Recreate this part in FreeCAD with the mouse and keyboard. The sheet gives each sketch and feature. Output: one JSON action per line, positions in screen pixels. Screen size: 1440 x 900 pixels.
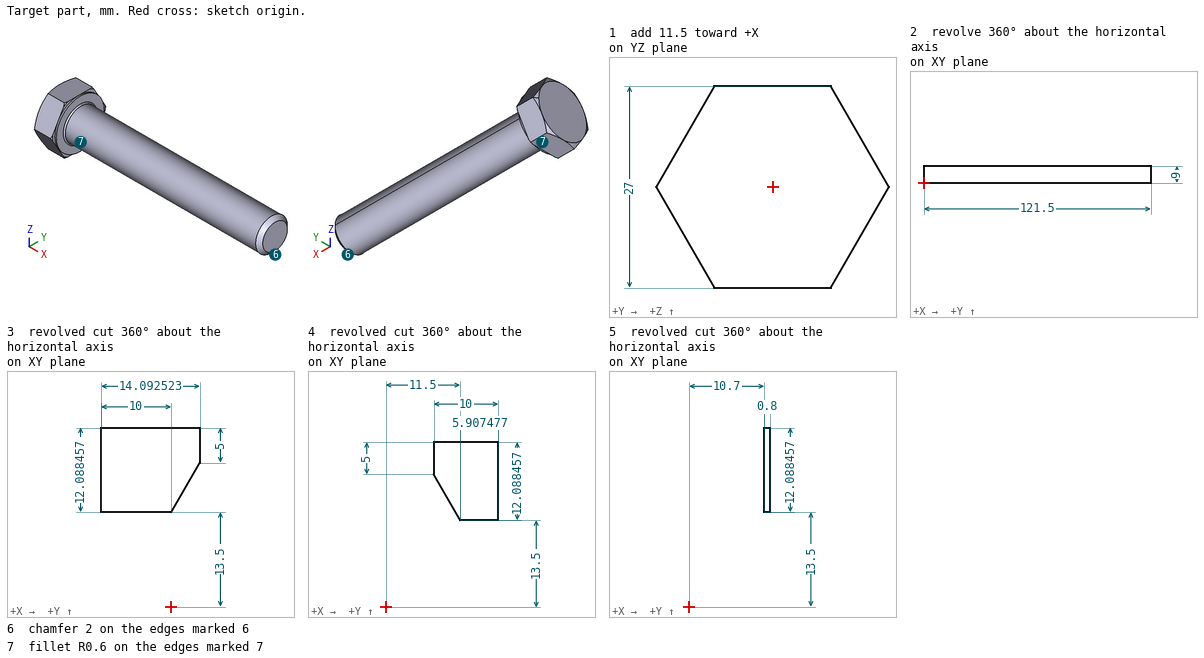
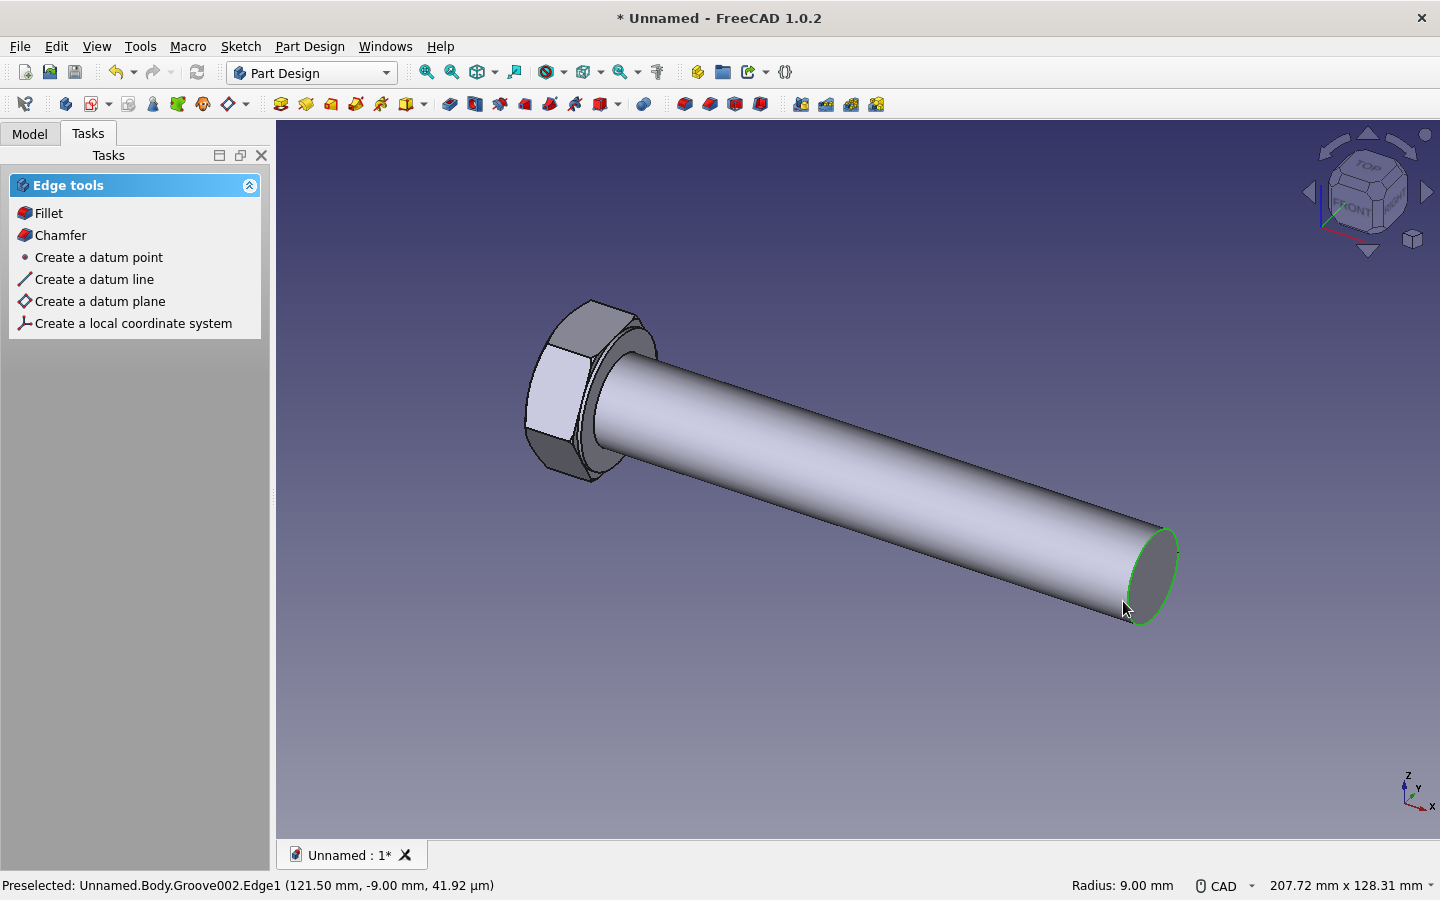
{"action": "left_click", "coordinate": [710, 104]}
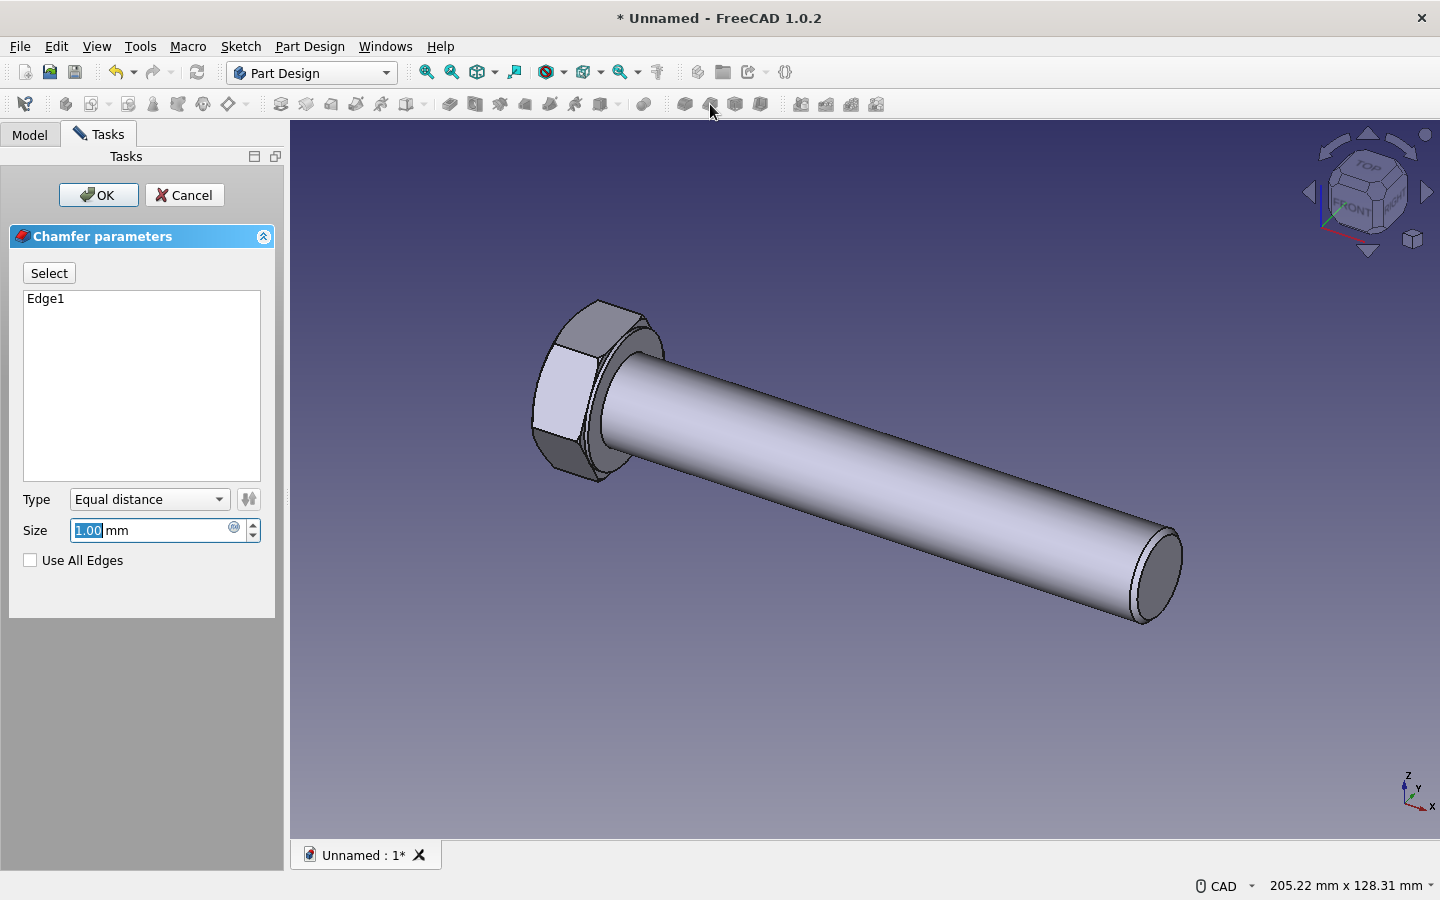
{"action": "type", "text": "2"}
{"action": "key", "text": "Tab"}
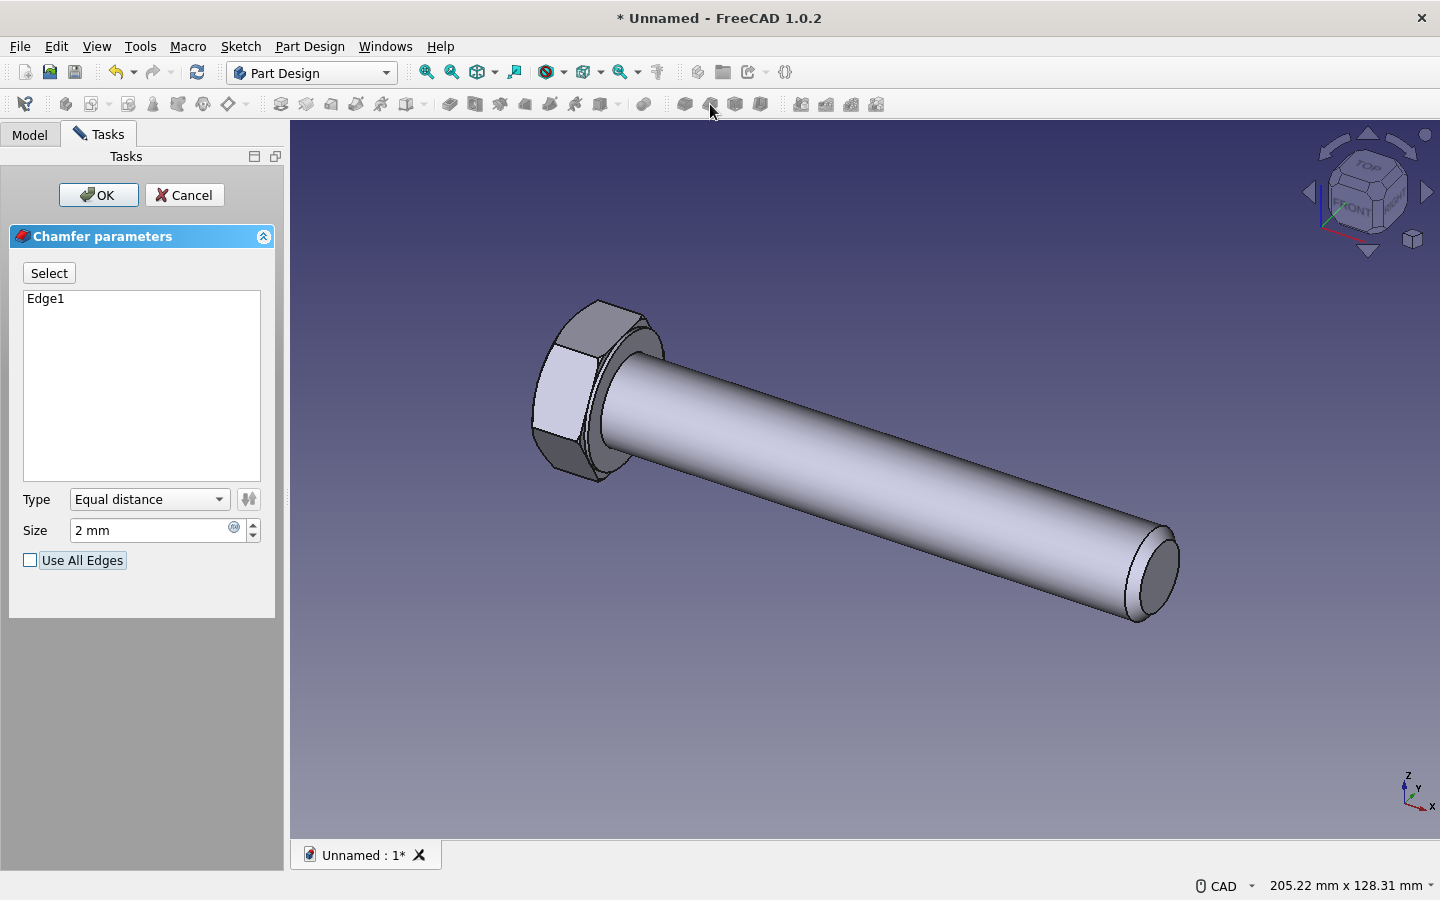
{"action": "left_click", "coordinate": [99, 195]}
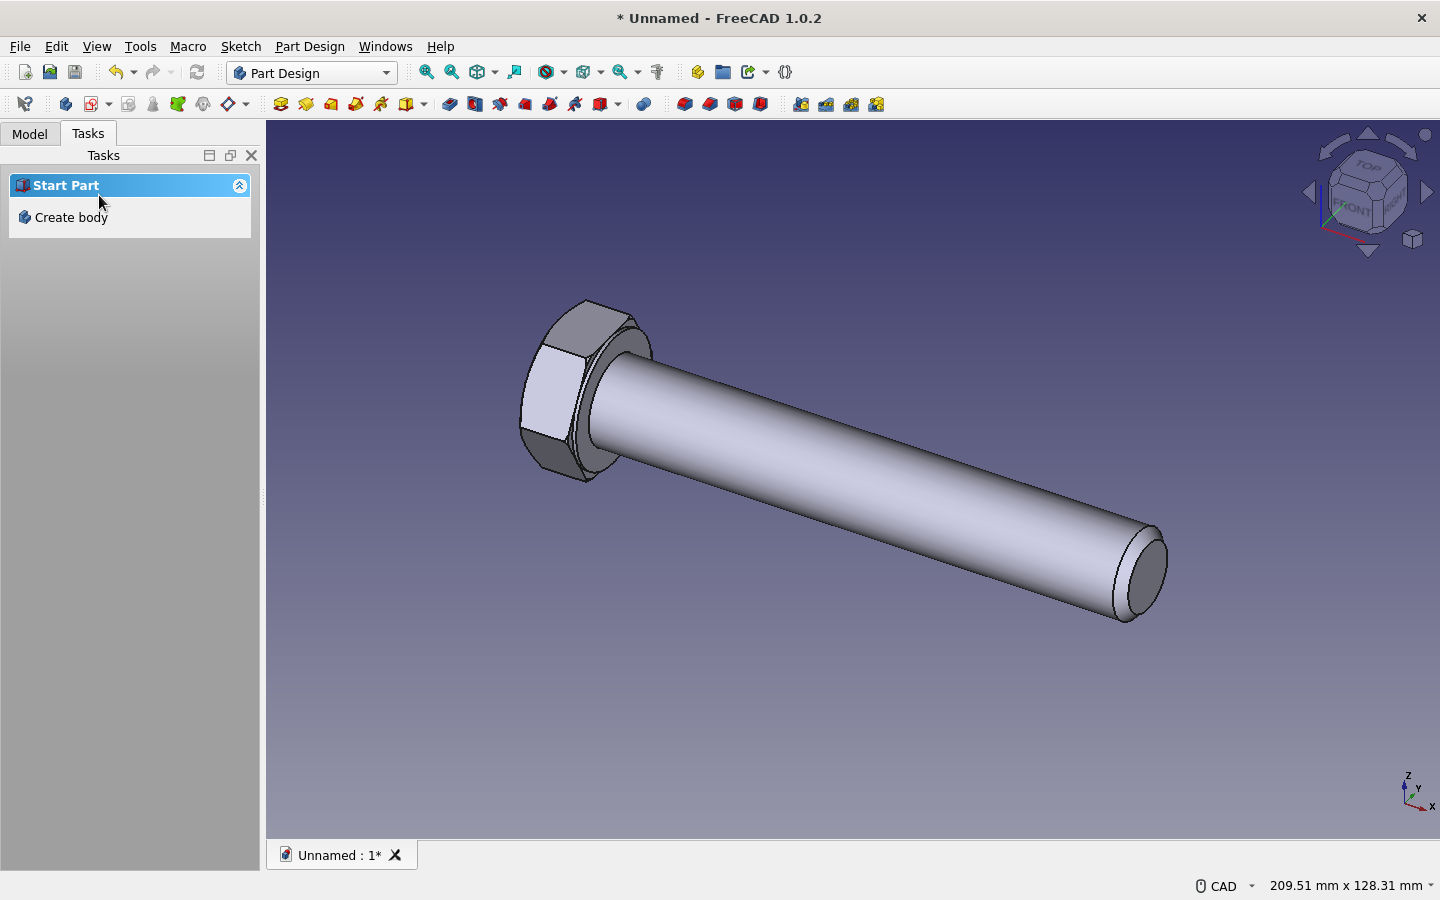
{"action": "key", "text": "0"}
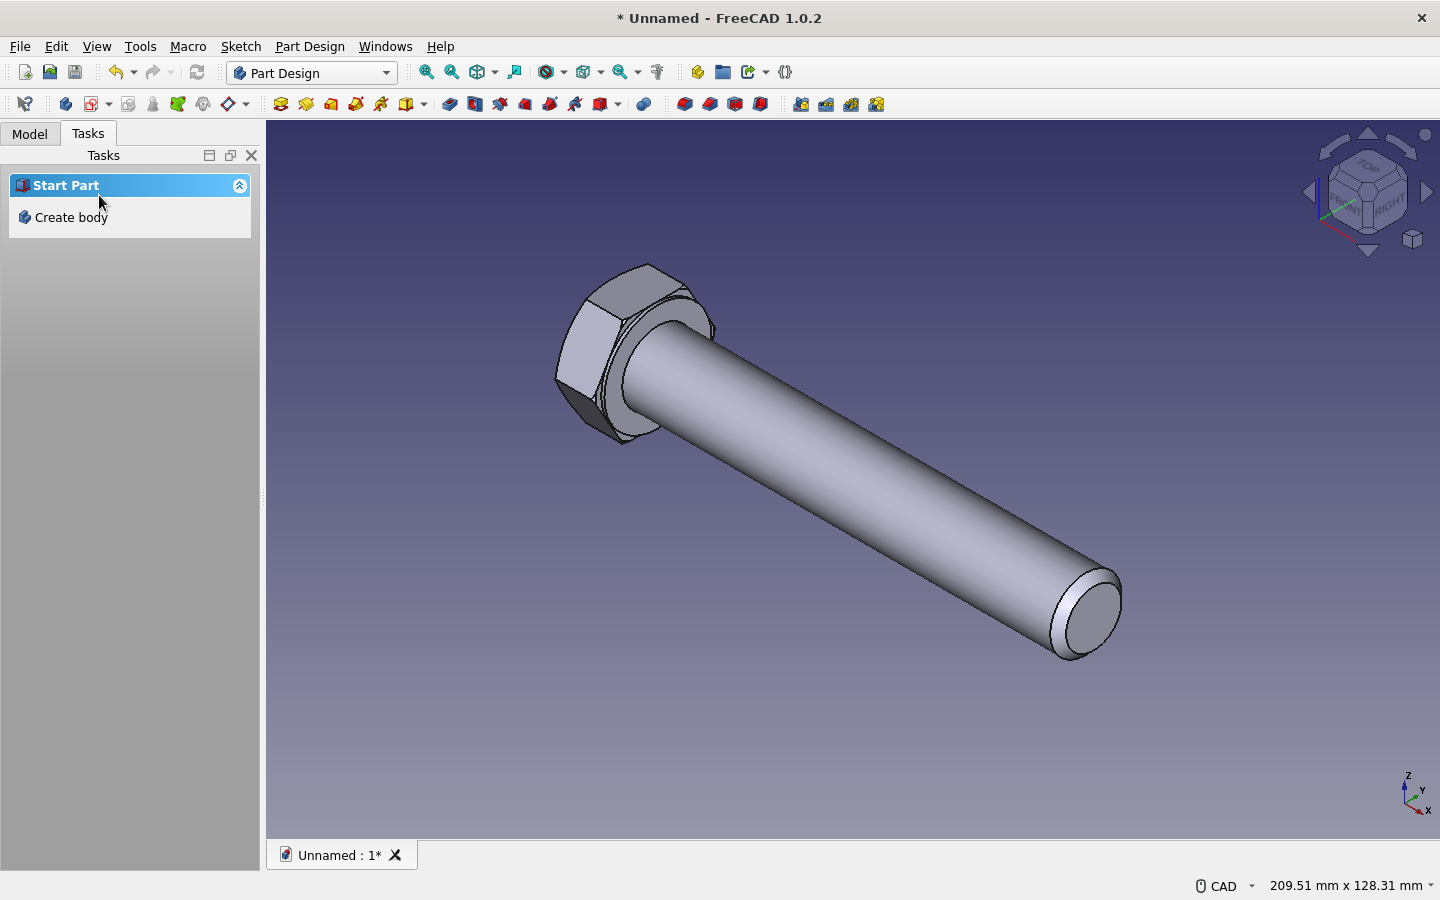
{"action": "key", "text": "2"}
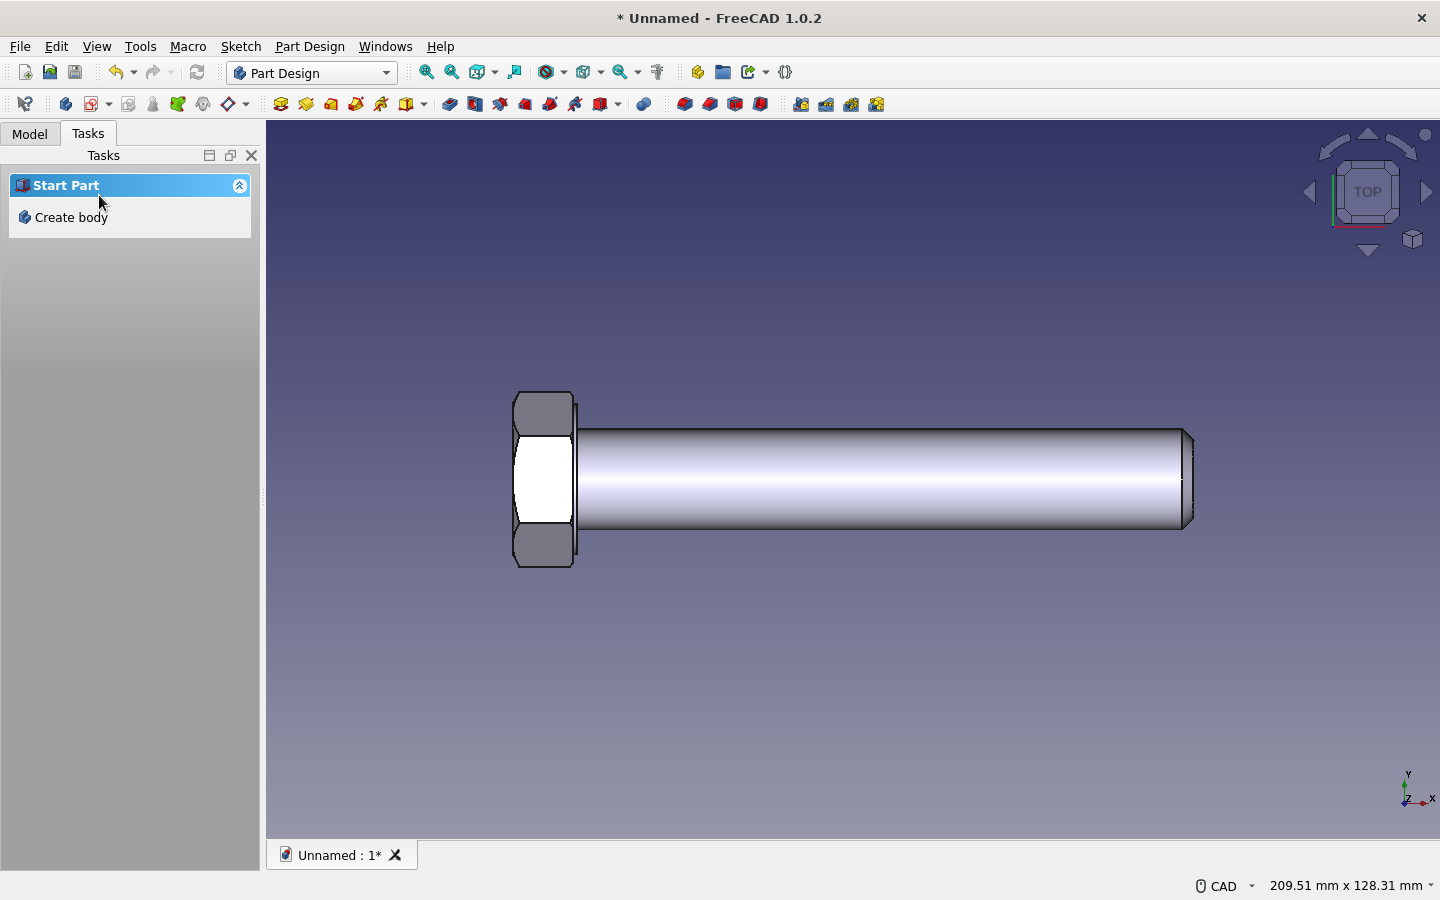
{"action": "key", "text": "1"}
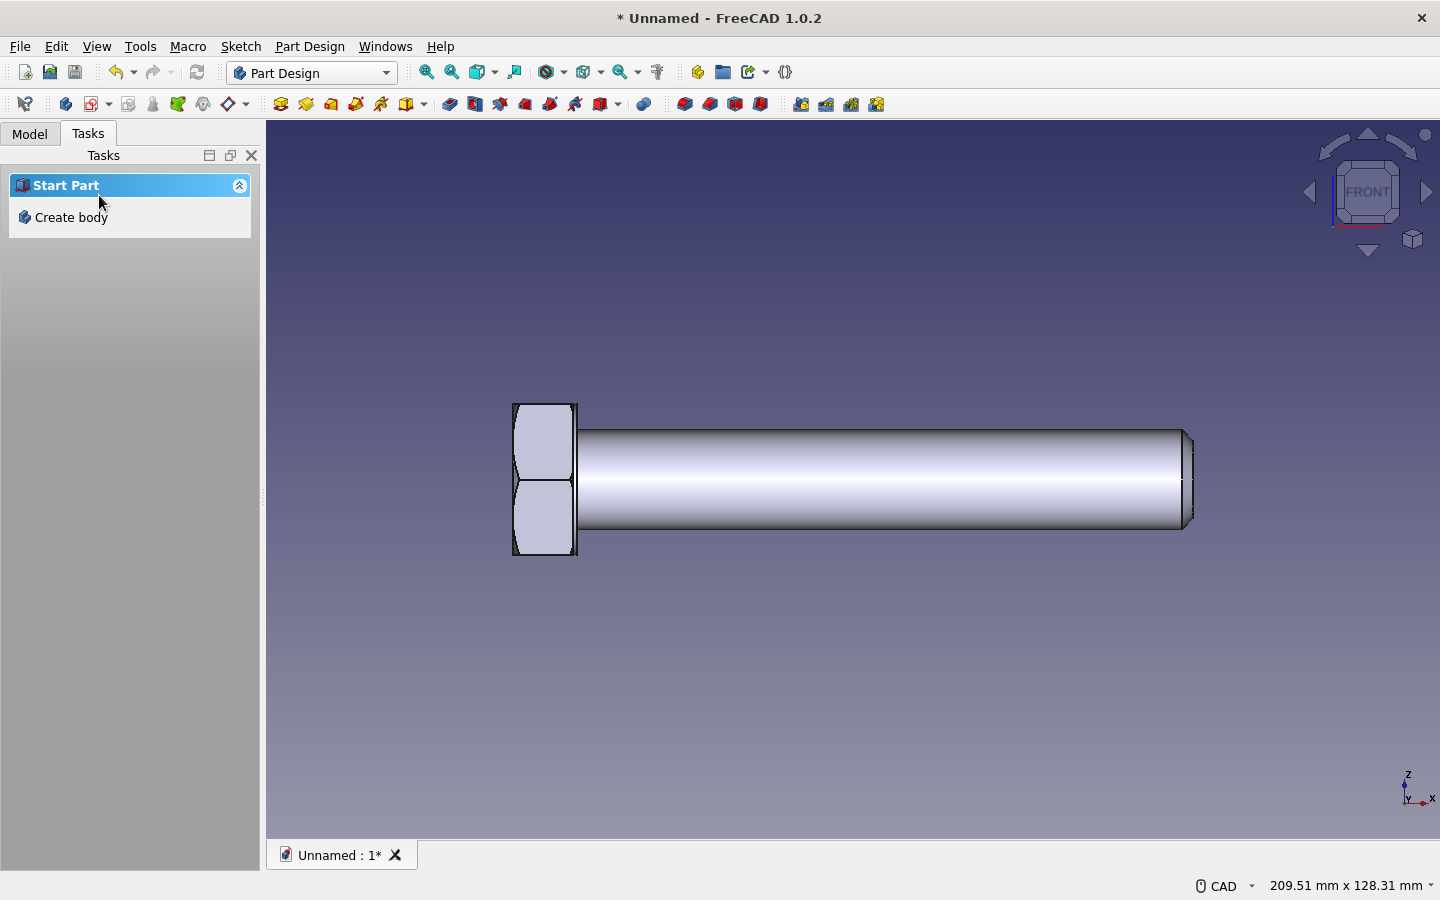
{"action": "key", "text": "3"}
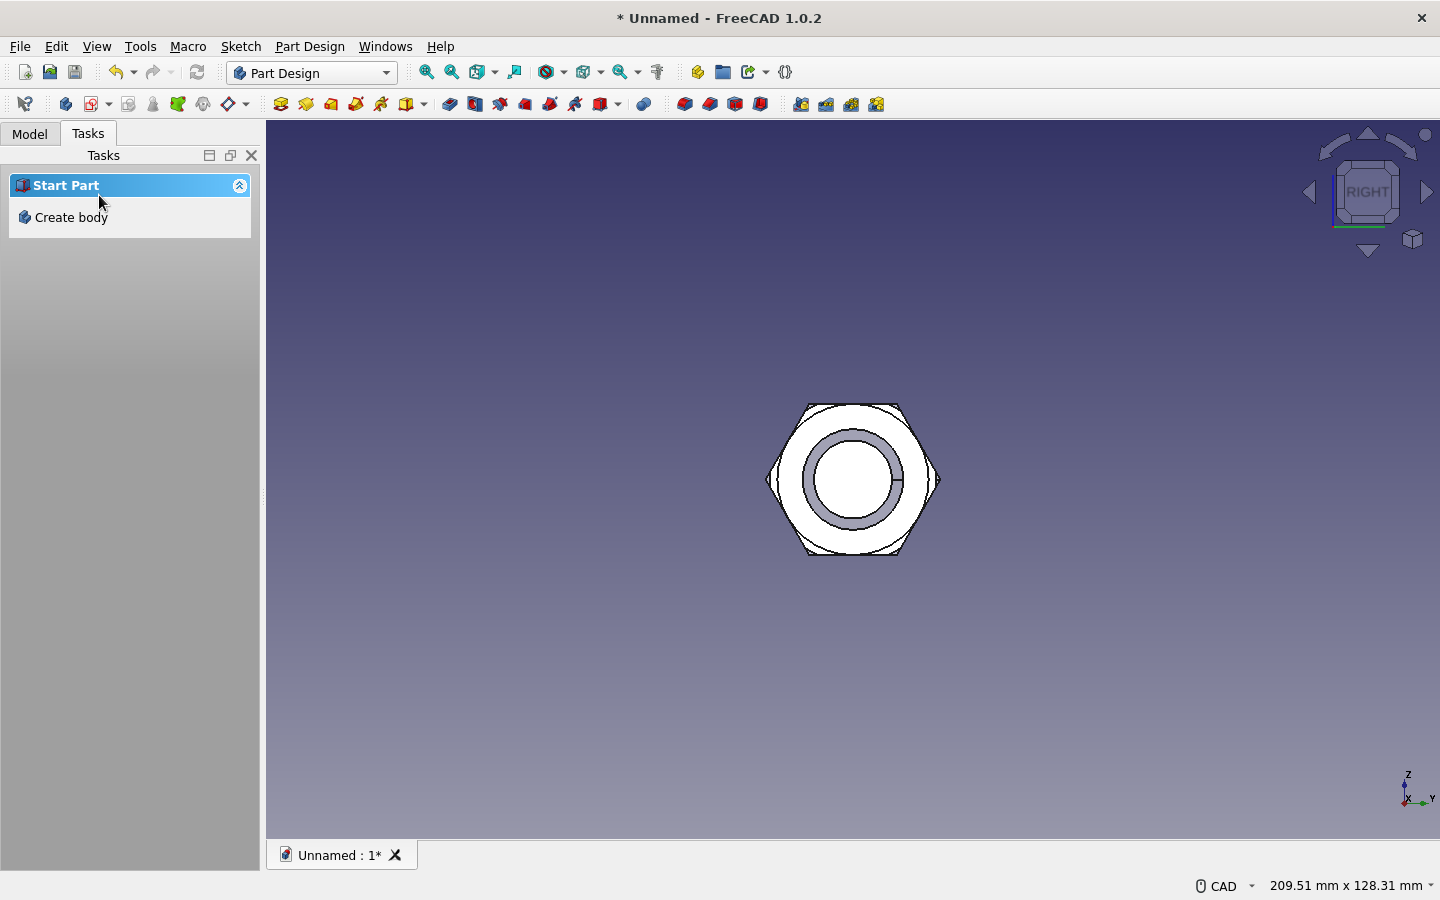
{"action": "left_click", "coordinate": [427, 72]}